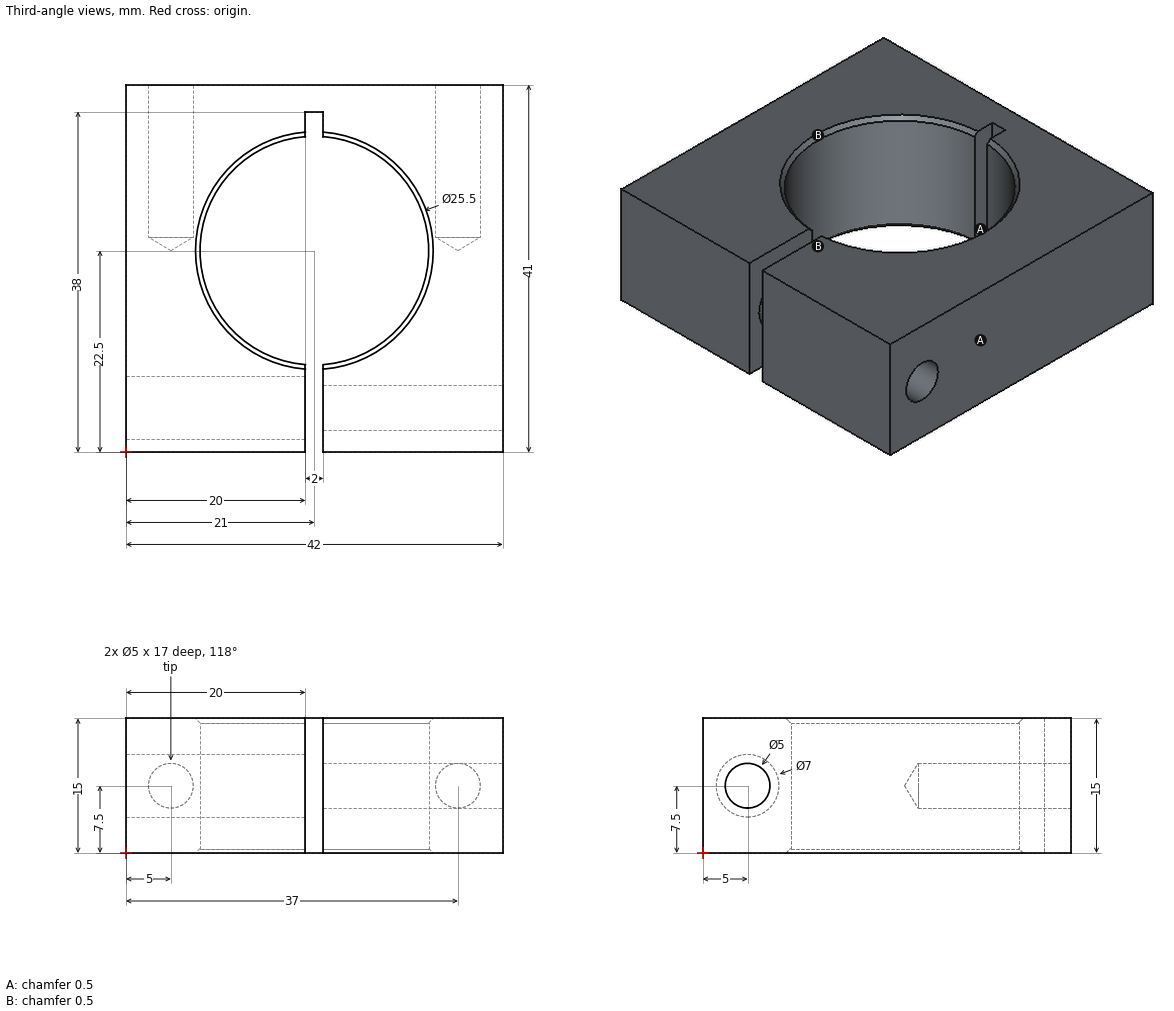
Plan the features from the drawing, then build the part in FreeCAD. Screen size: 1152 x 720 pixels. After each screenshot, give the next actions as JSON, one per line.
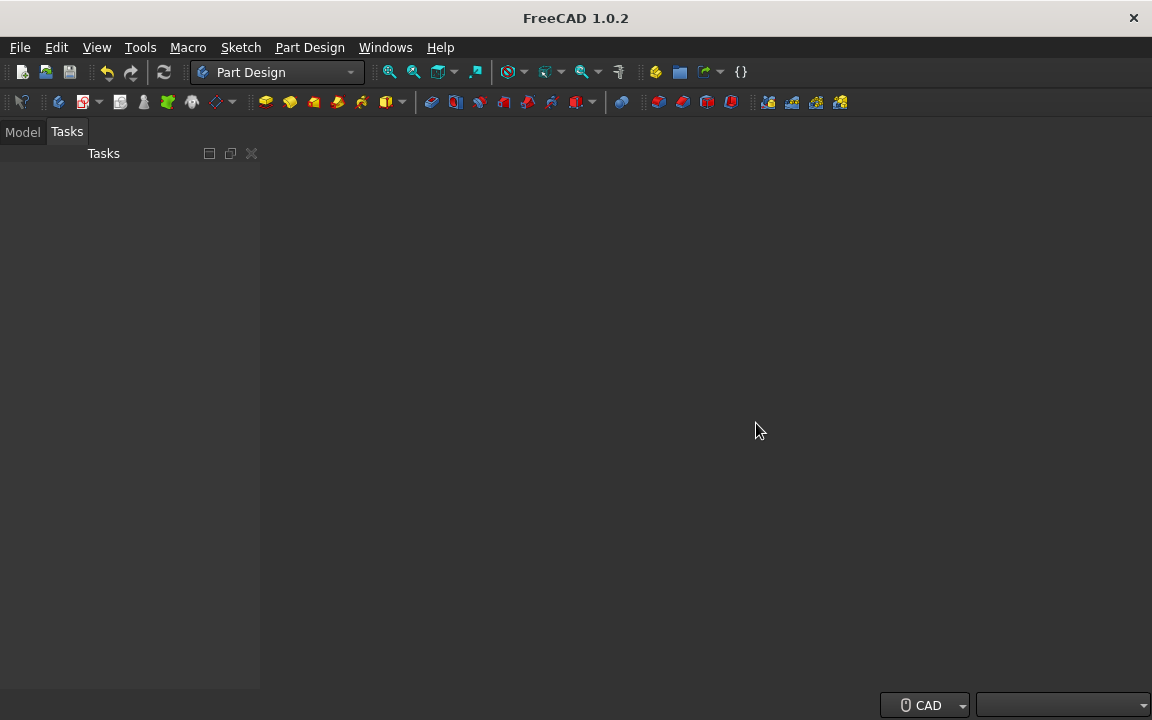
{"action": "left_click", "coordinate": [22, 72]}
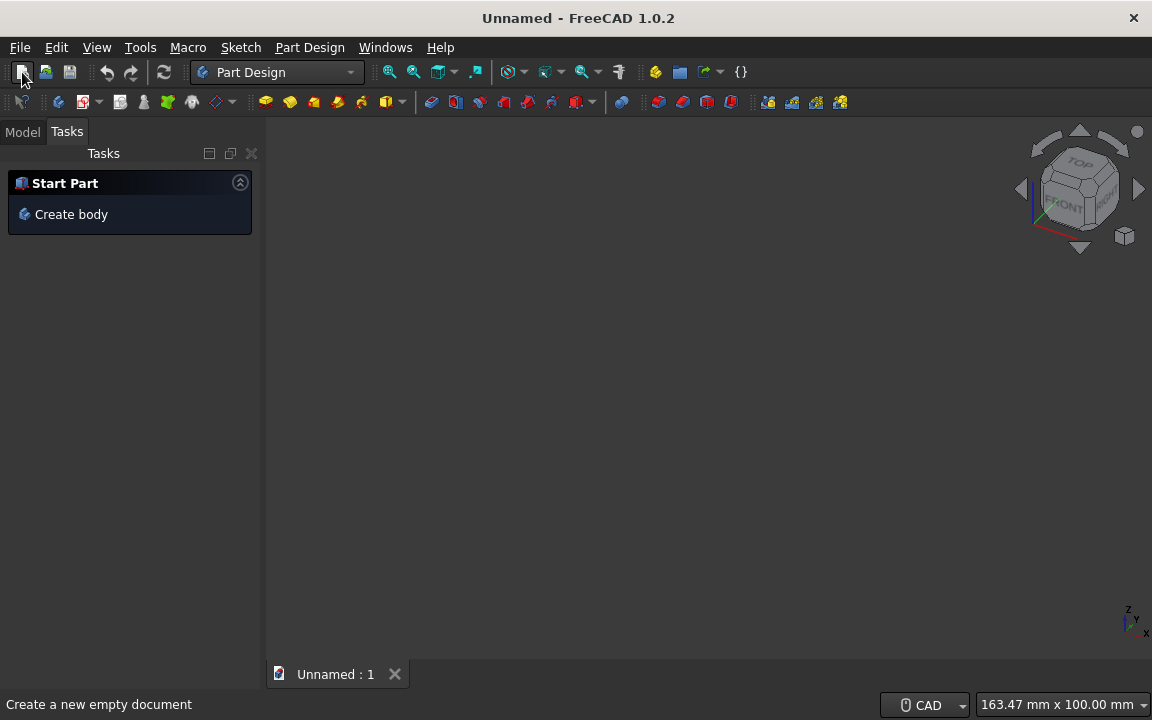
{"action": "left_click", "coordinate": [84, 102]}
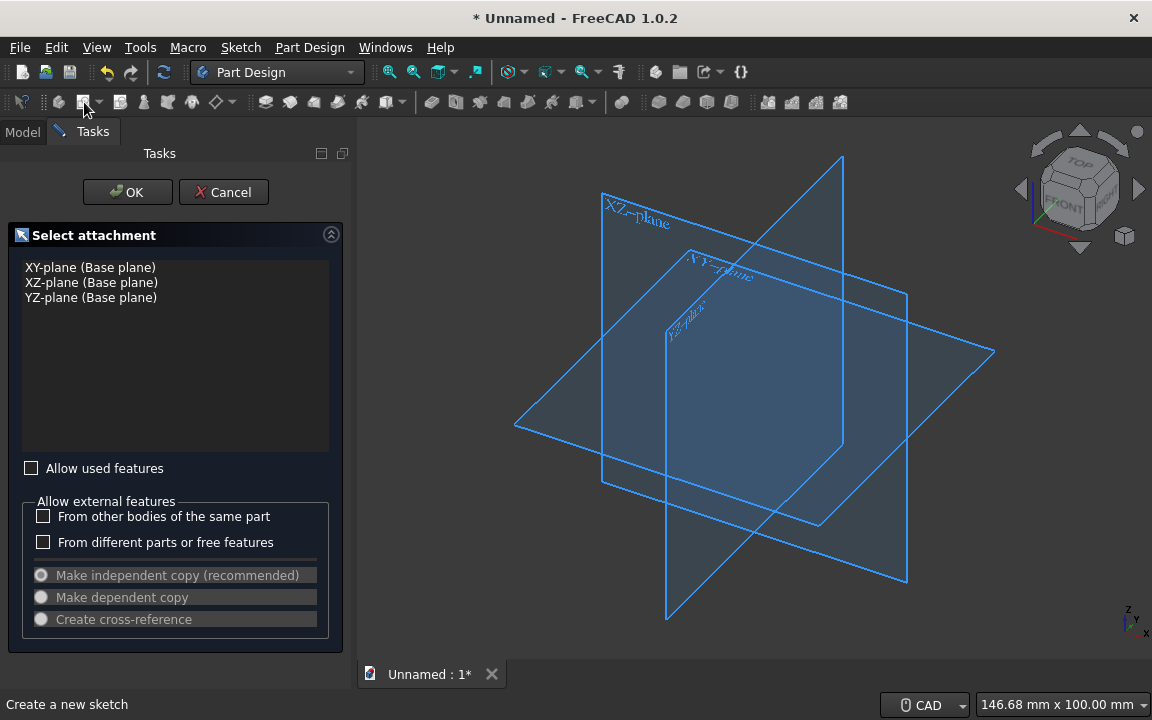
{"action": "left_click", "coordinate": [82, 268]}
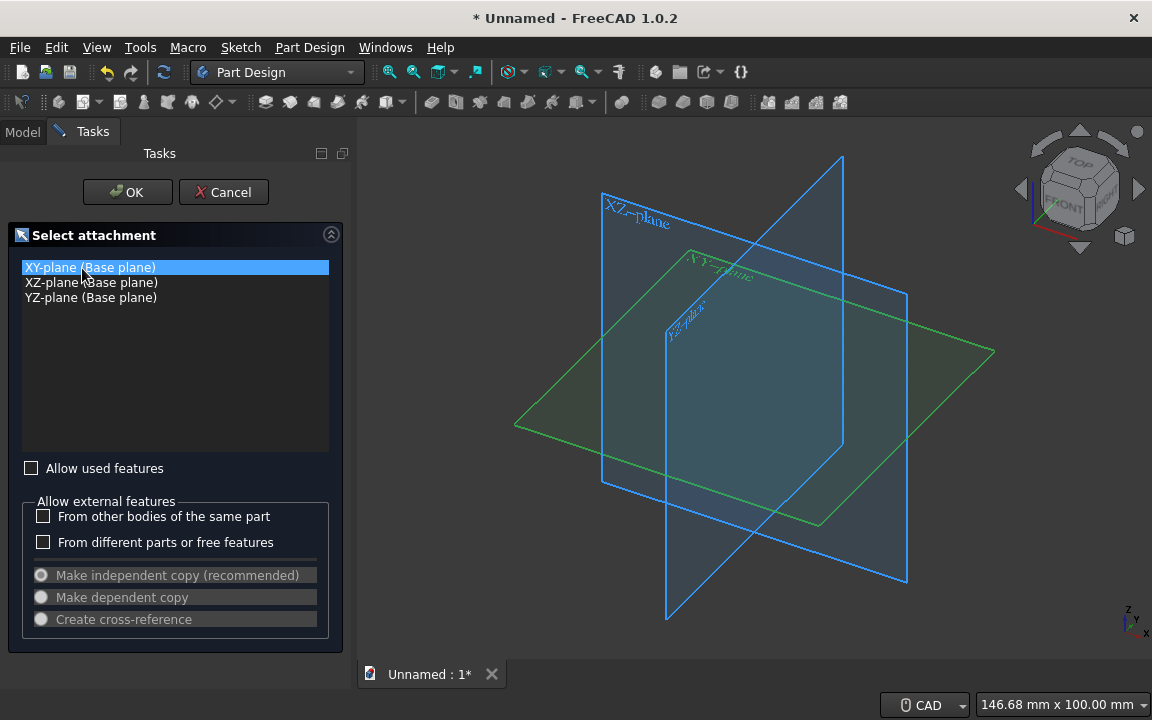
{"action": "left_click", "coordinate": [128, 192]}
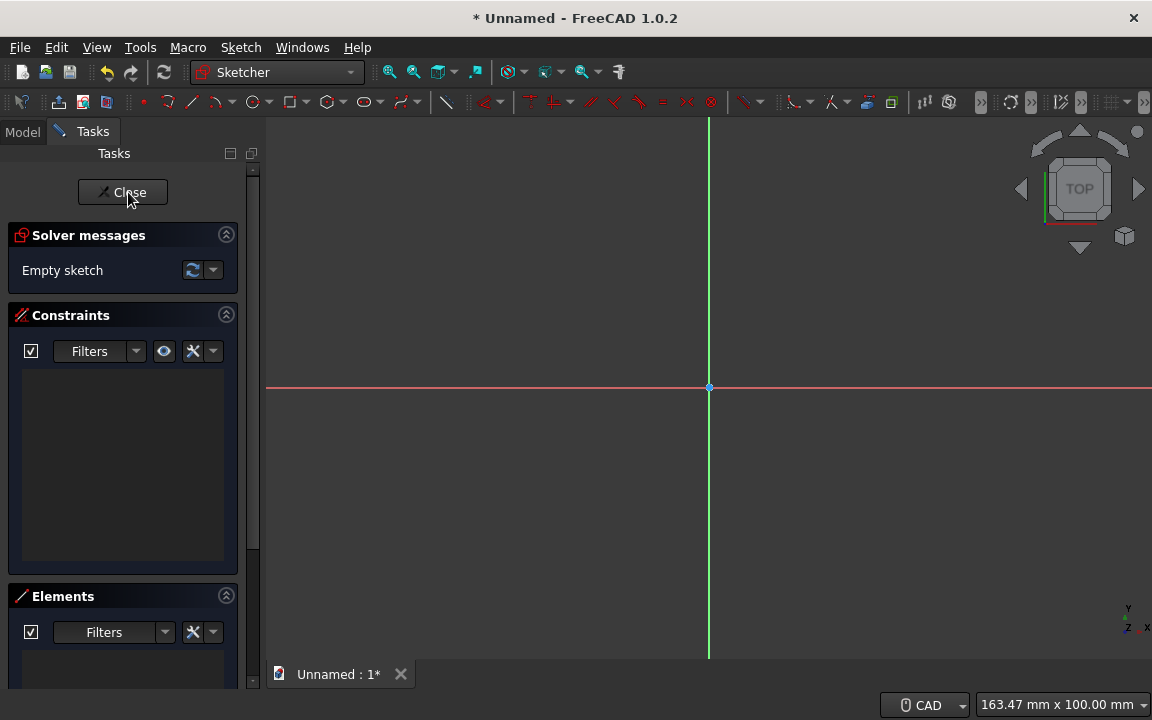
{"action": "scroll", "coordinate": [987, 145], "scroll_direction": "up", "scroll_amount": 2}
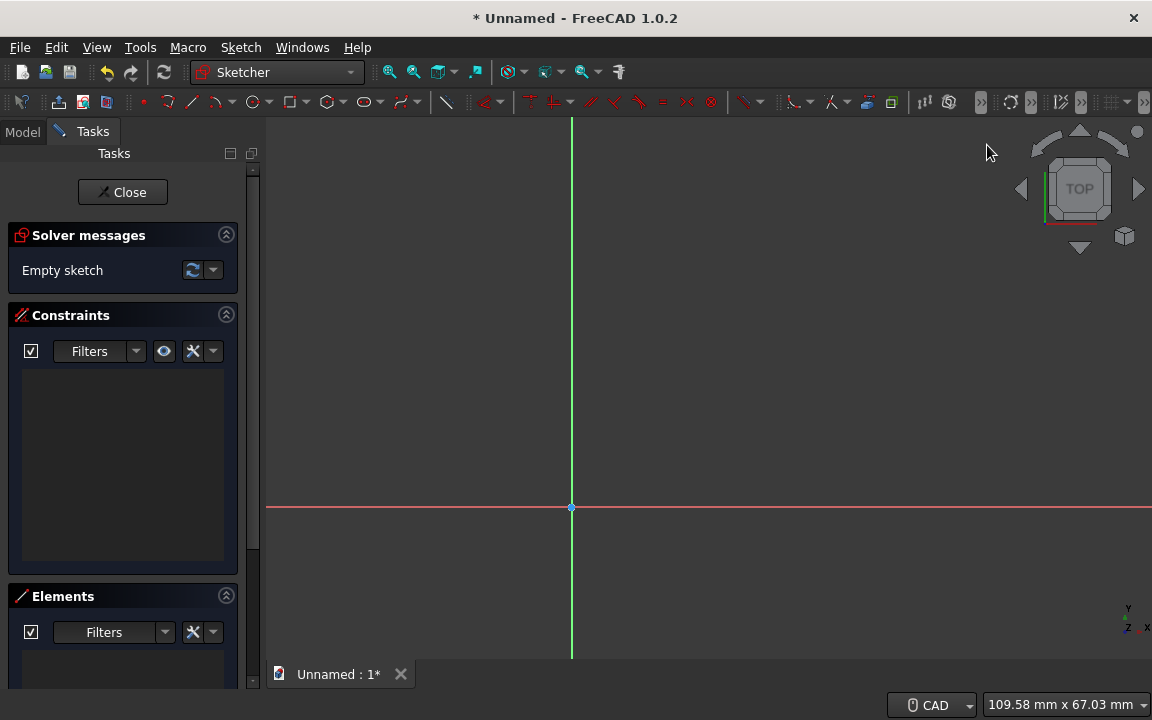
{"action": "left_click", "coordinate": [290, 102]}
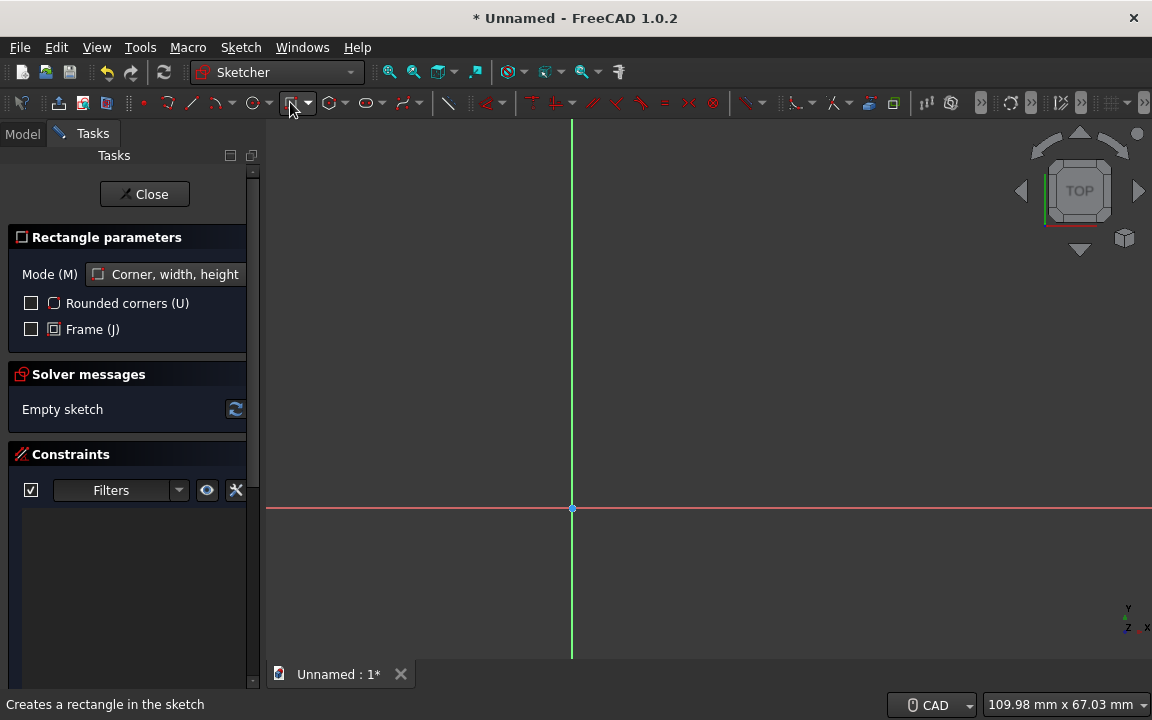
{"action": "left_click", "coordinate": [572, 508]}
{"action": "mouse_move", "coordinate": [911, 178]}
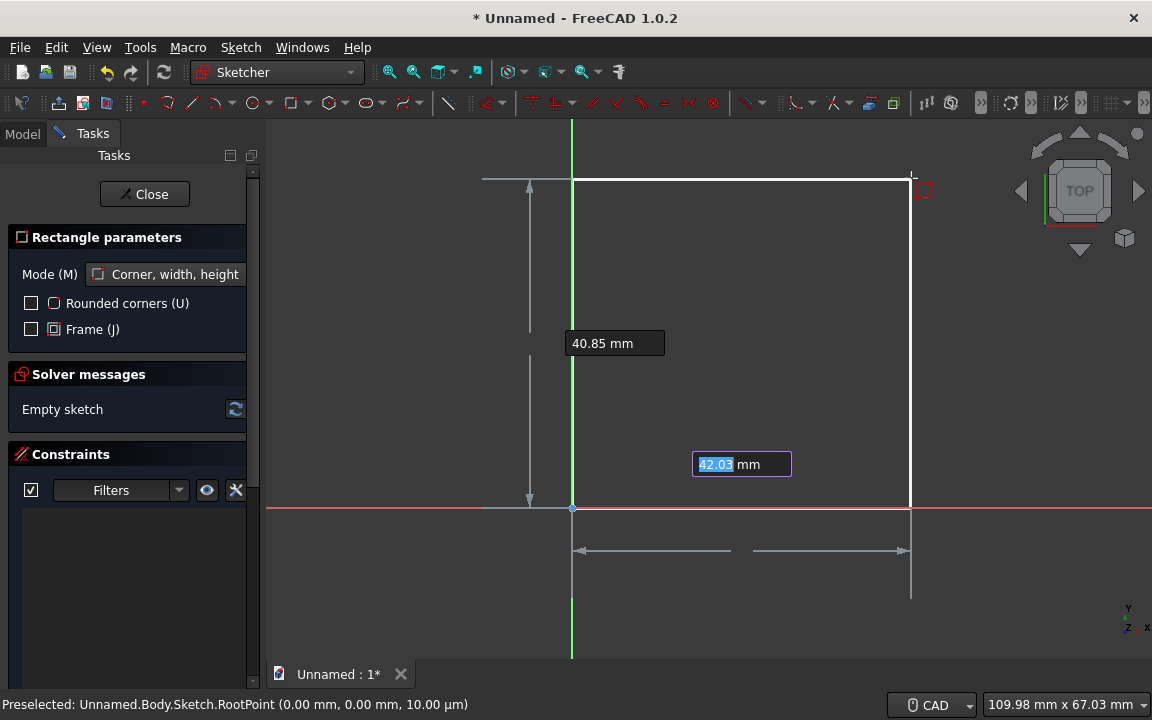
{"action": "type", "text": "42"}
{"action": "key", "text": "Tab"}
{"action": "type", "text": "41"}
{"action": "key", "text": "Return"}
{"action": "key", "text": "Escape"}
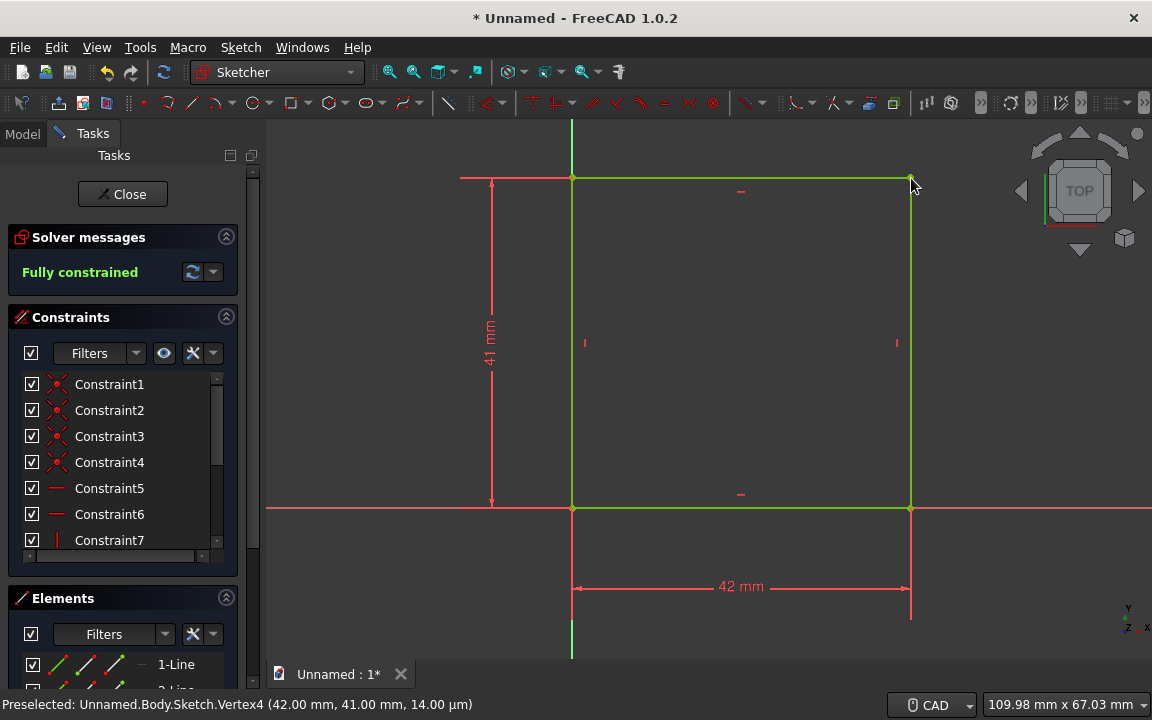
{"action": "left_click", "coordinate": [123, 194]}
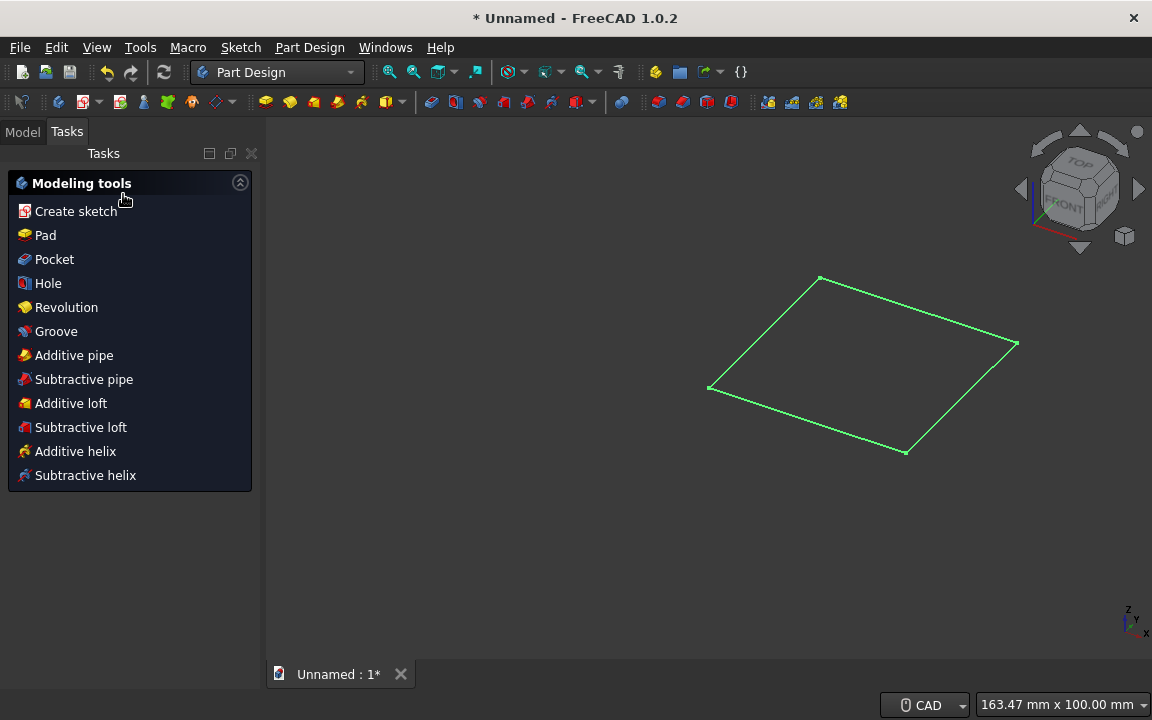
{"action": "left_click", "coordinate": [266, 102]}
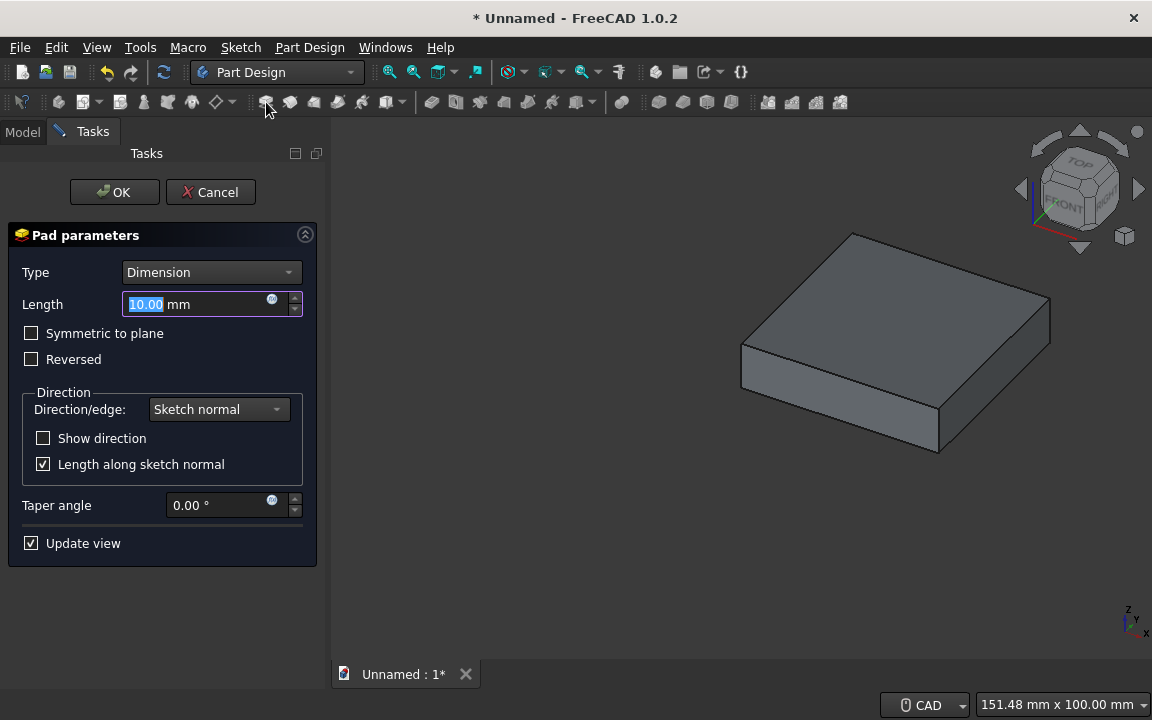
{"action": "type", "text": "15"}
{"action": "key", "text": "Tab"}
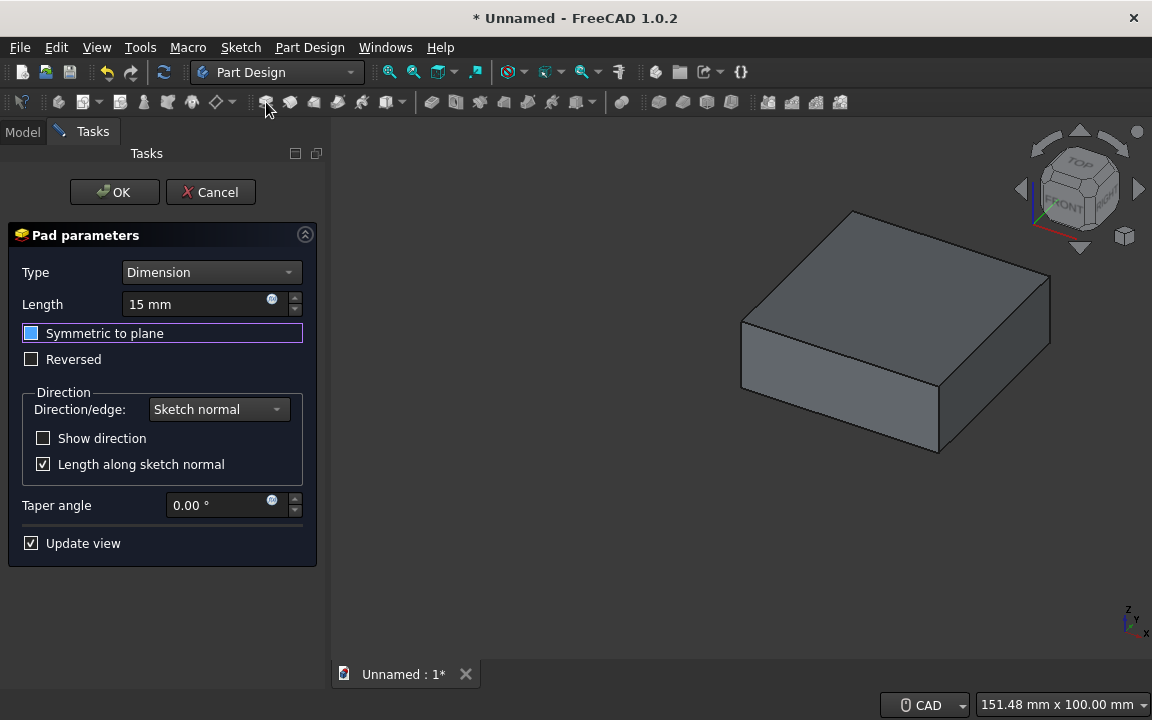
{"action": "left_click", "coordinate": [115, 192]}